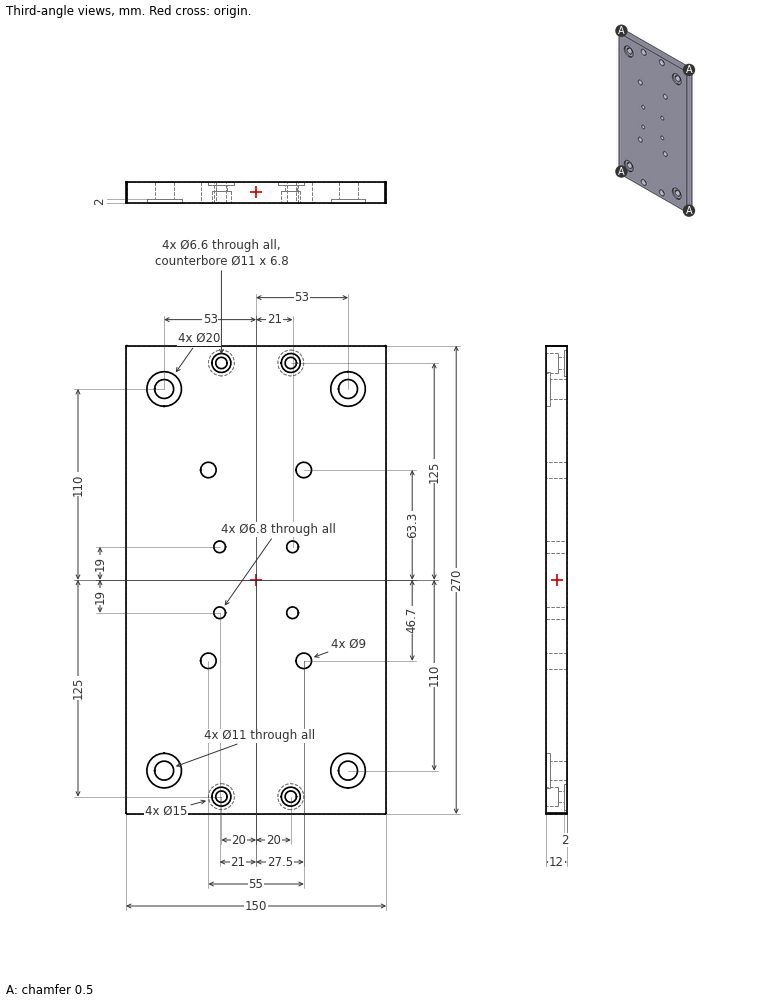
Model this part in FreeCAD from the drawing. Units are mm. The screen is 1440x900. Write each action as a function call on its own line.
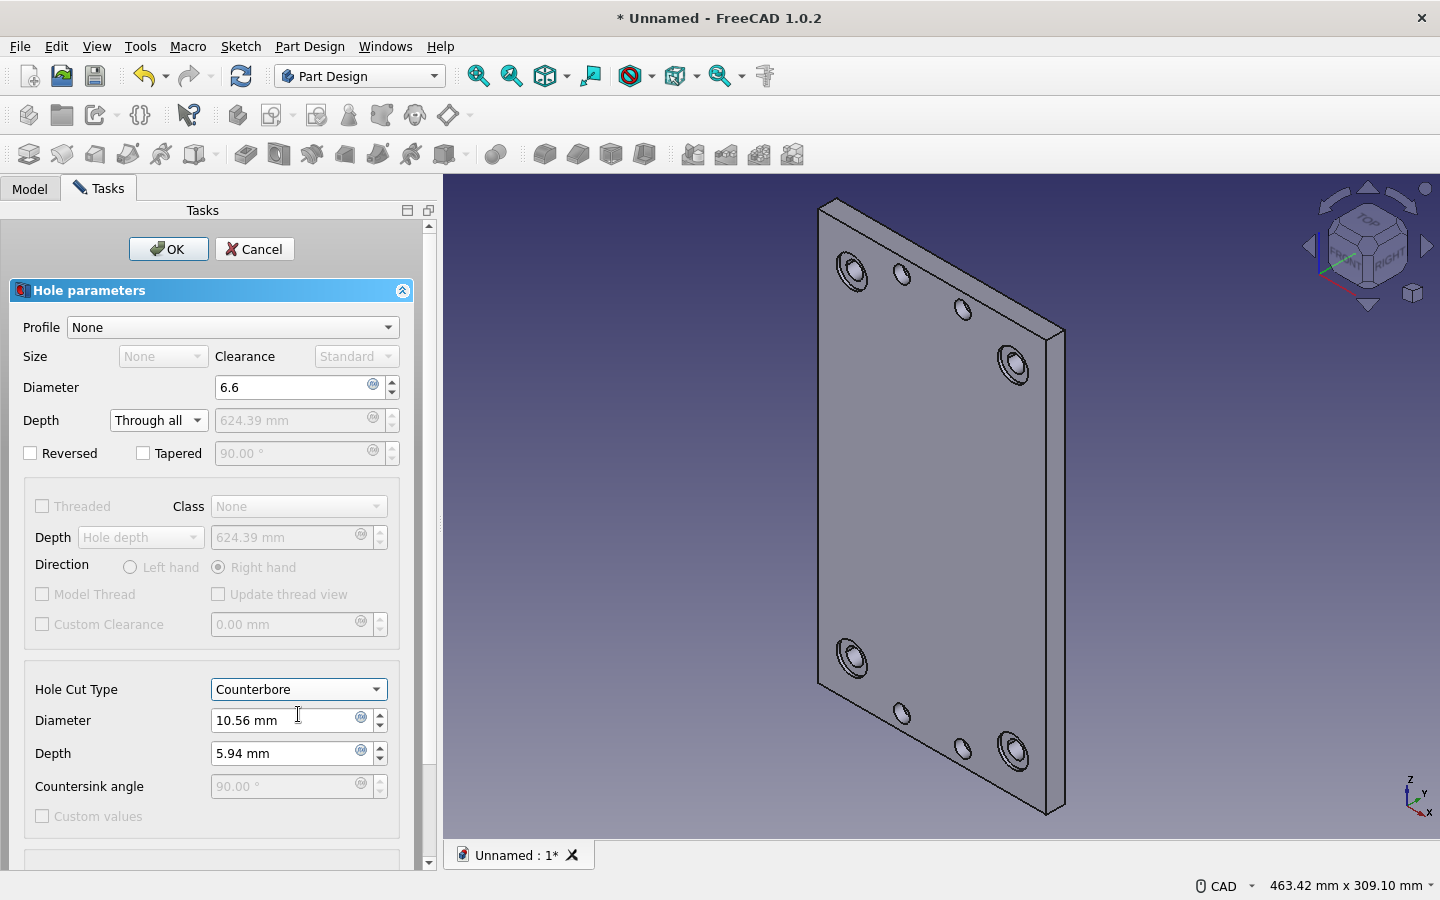
triple_click(292, 720)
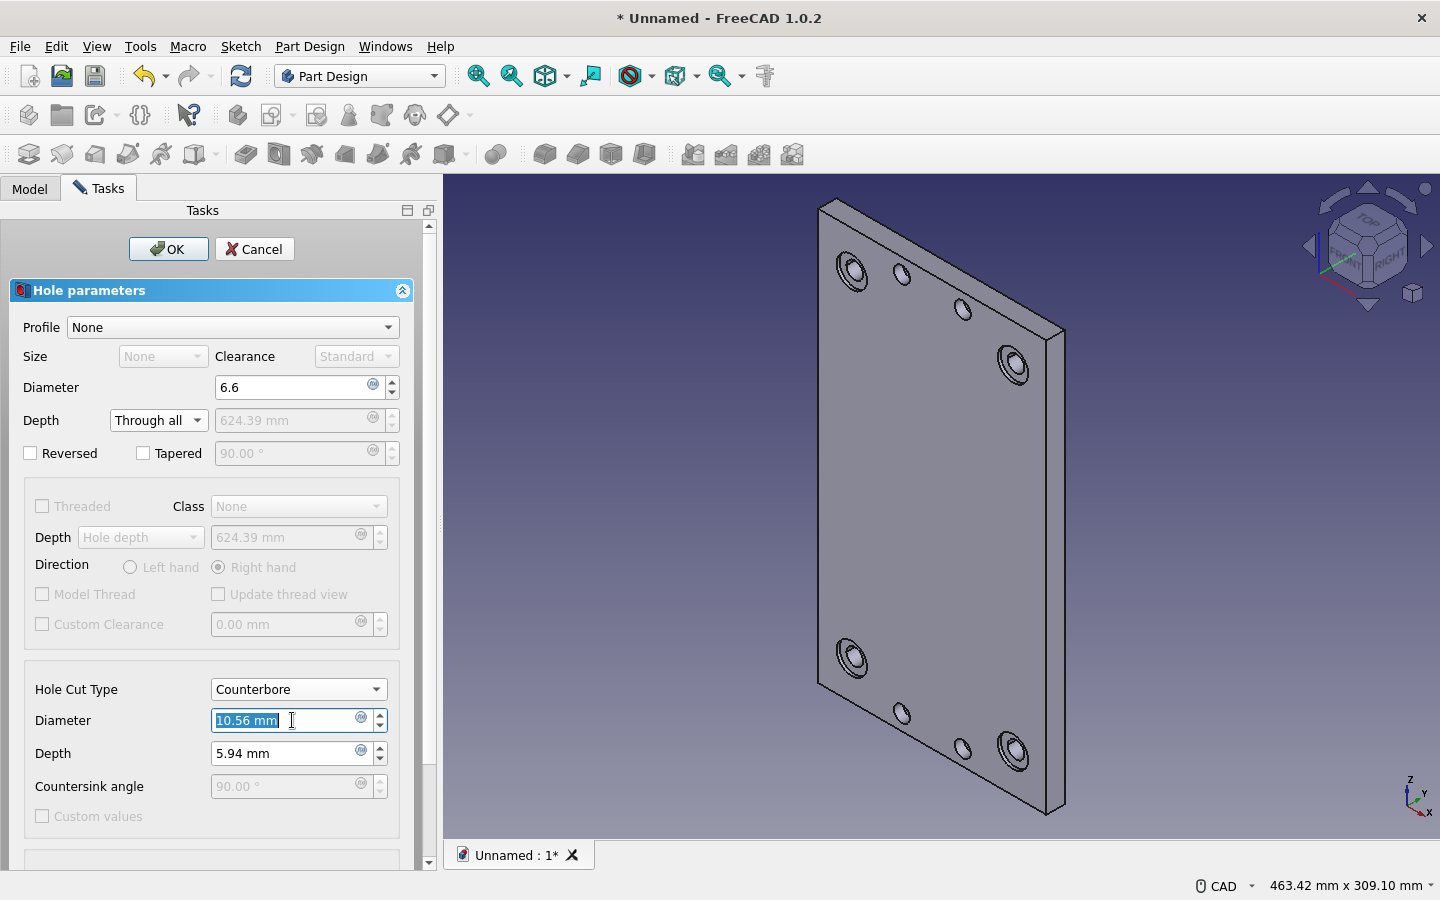
text(11)
key(Tab)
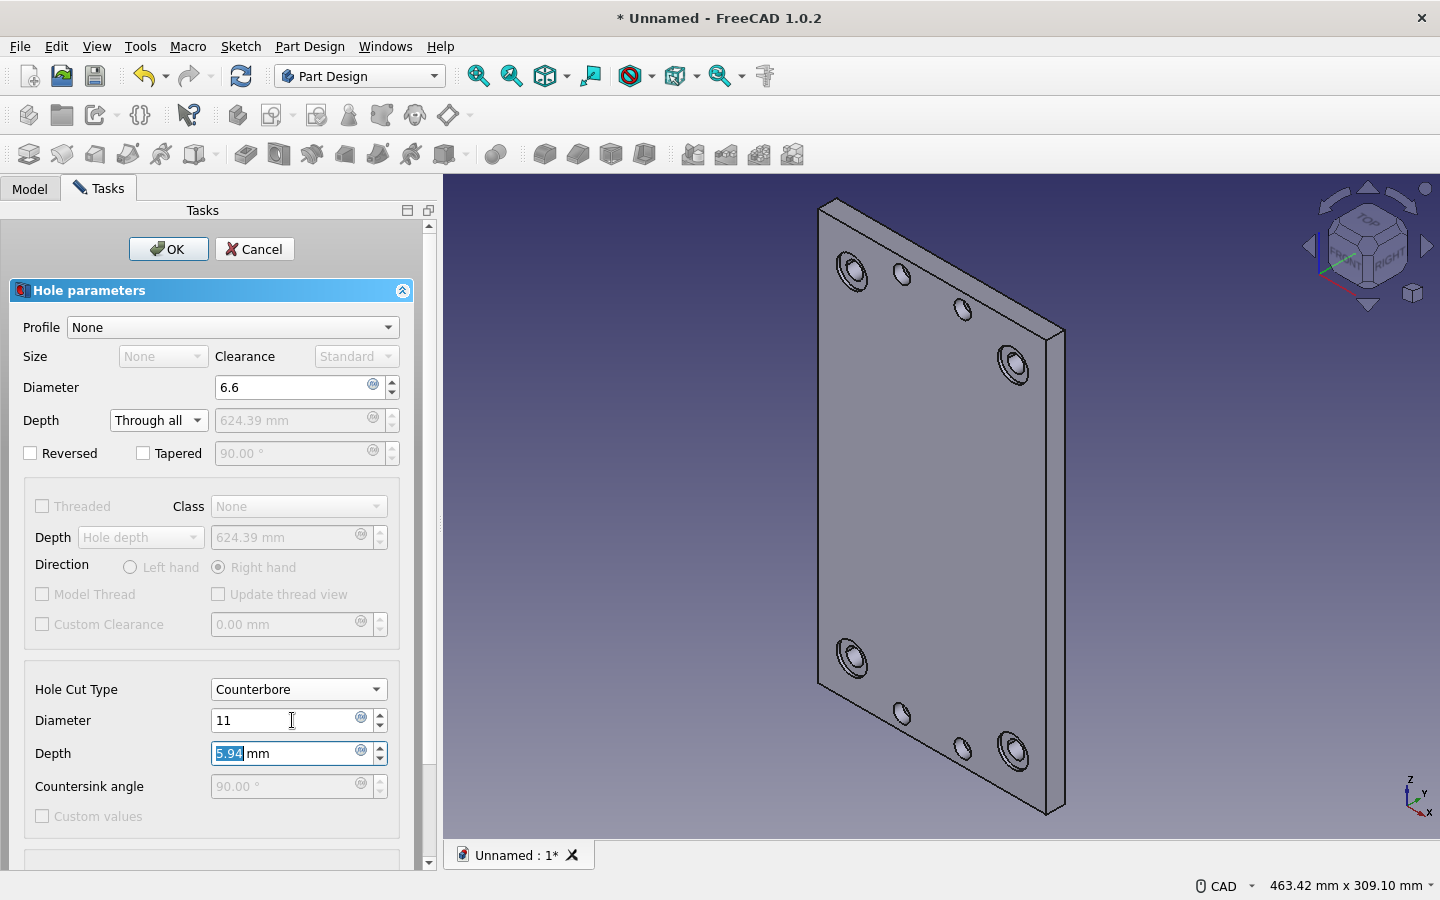
text(6.8)
key(Tab)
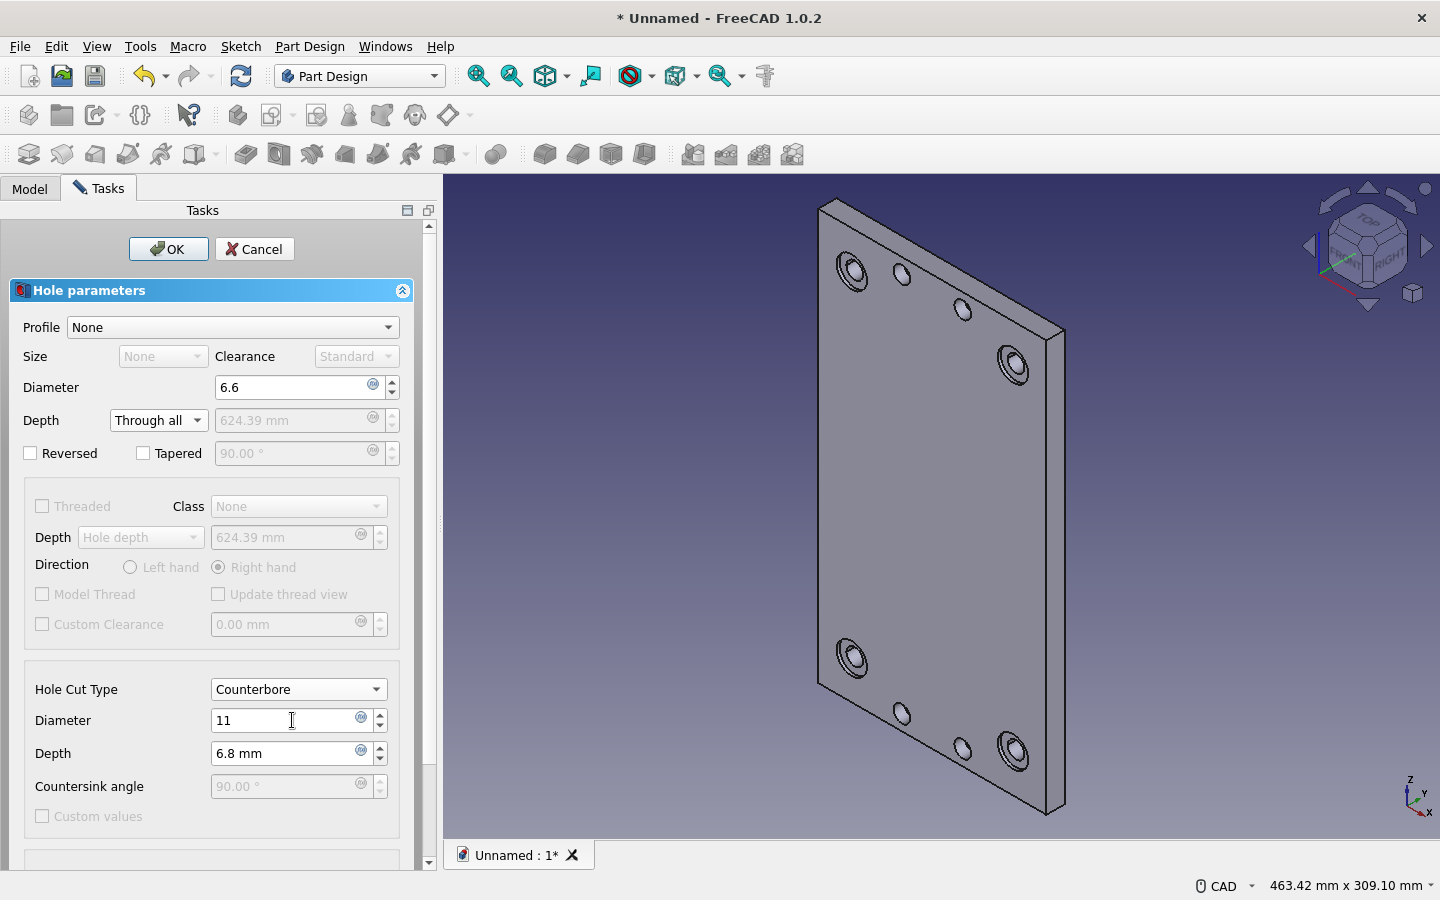
click(169, 249)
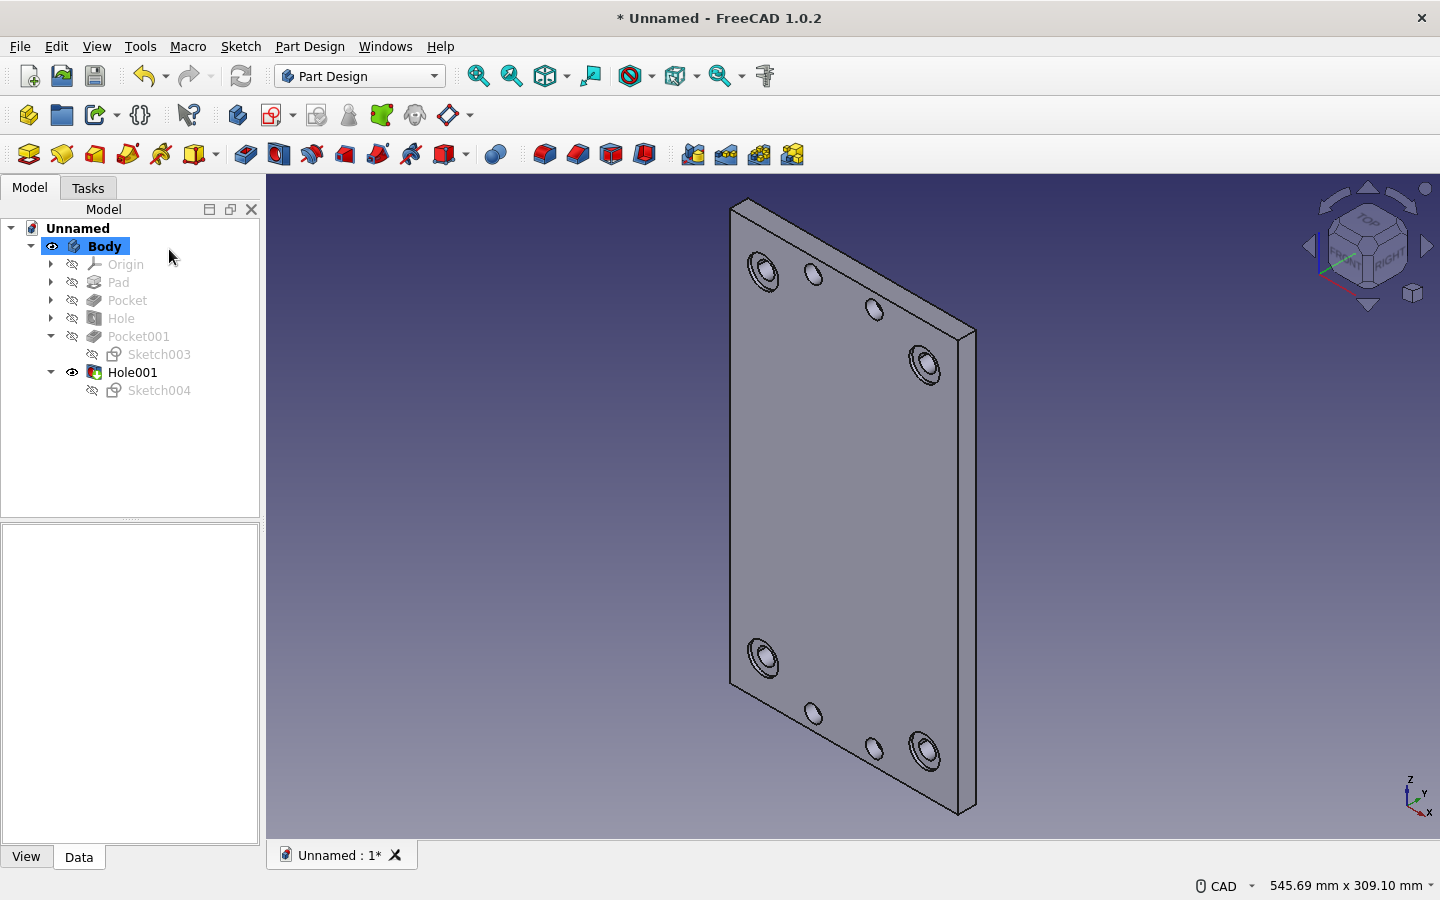
click(844, 443)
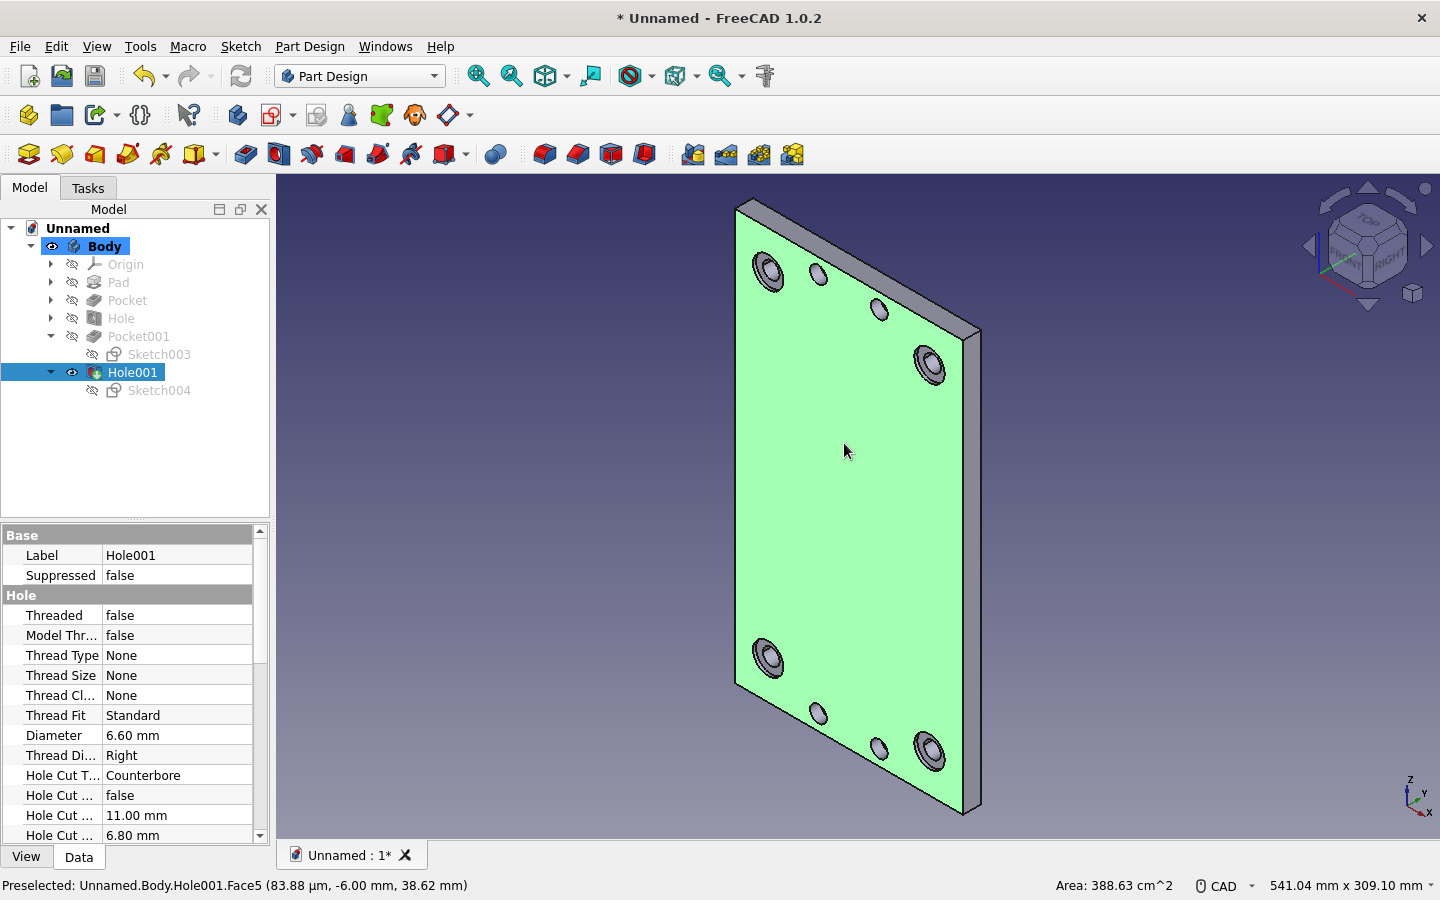
click(270, 116)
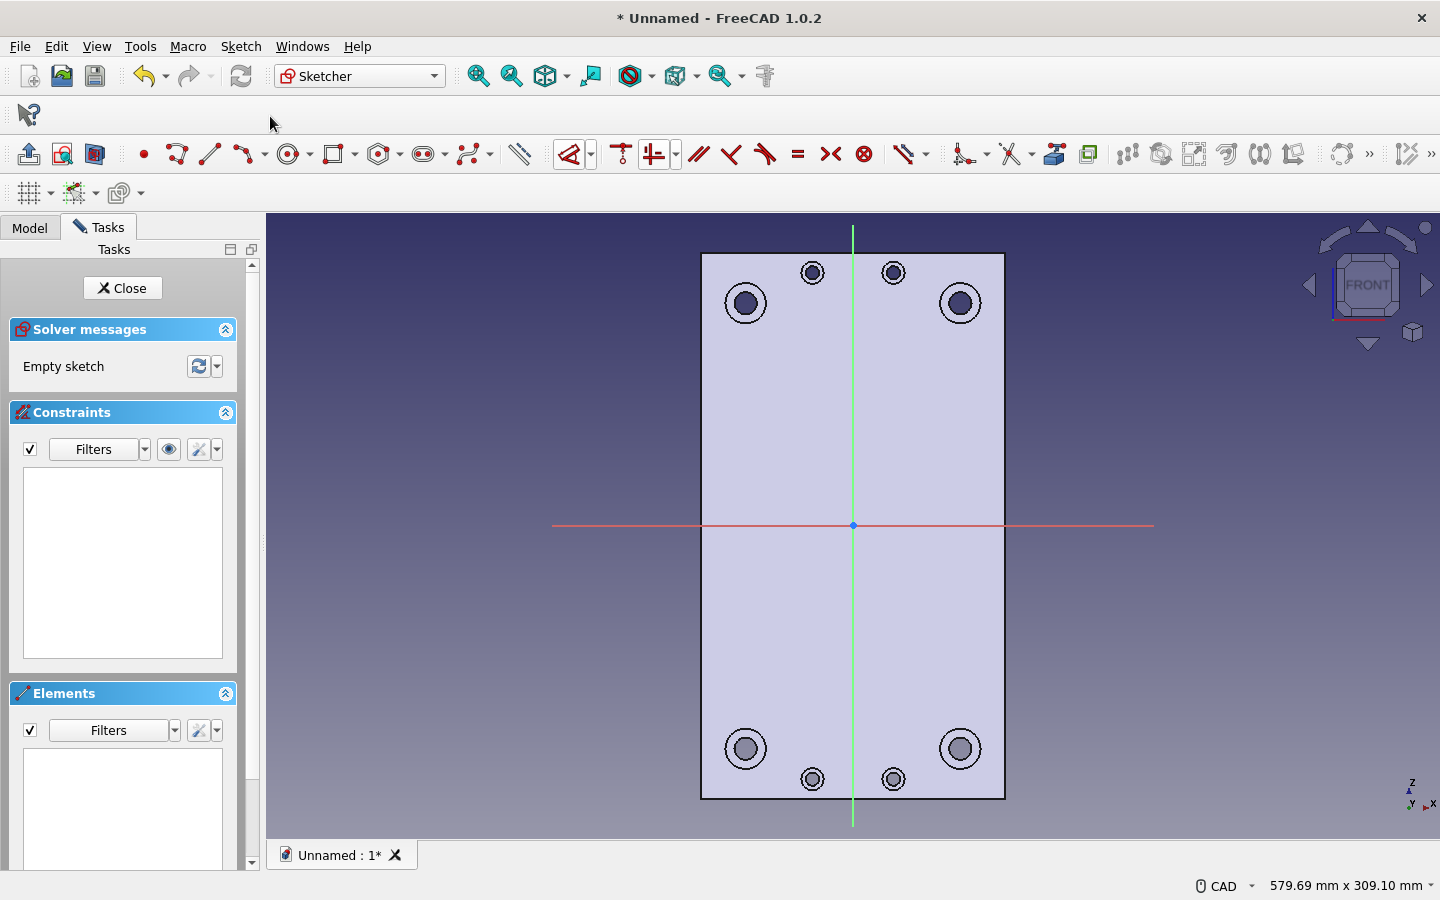
scroll(875, 526, up, 7)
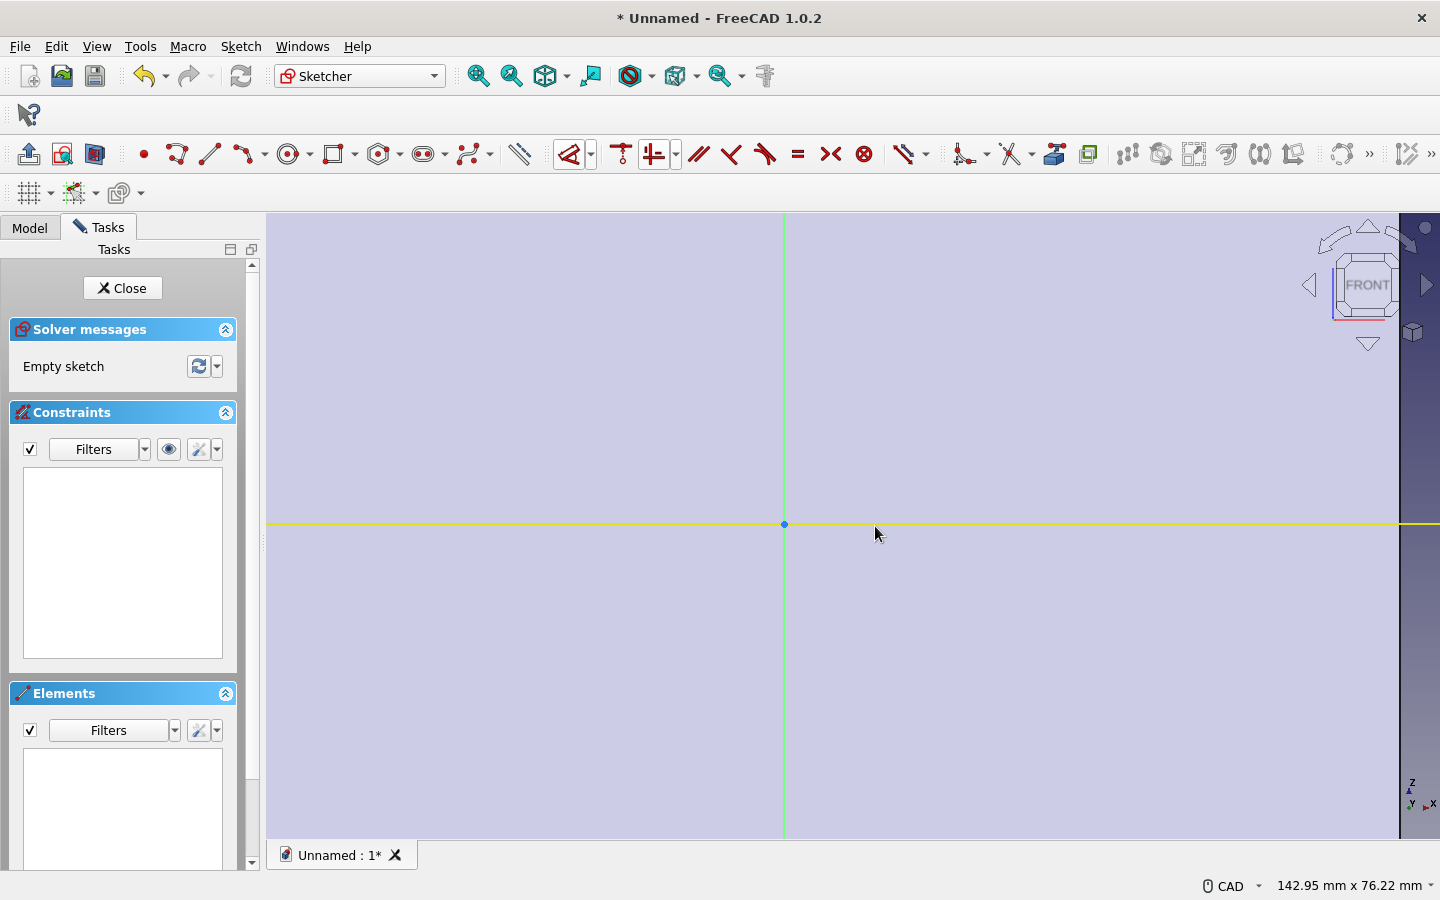
click(288, 154)